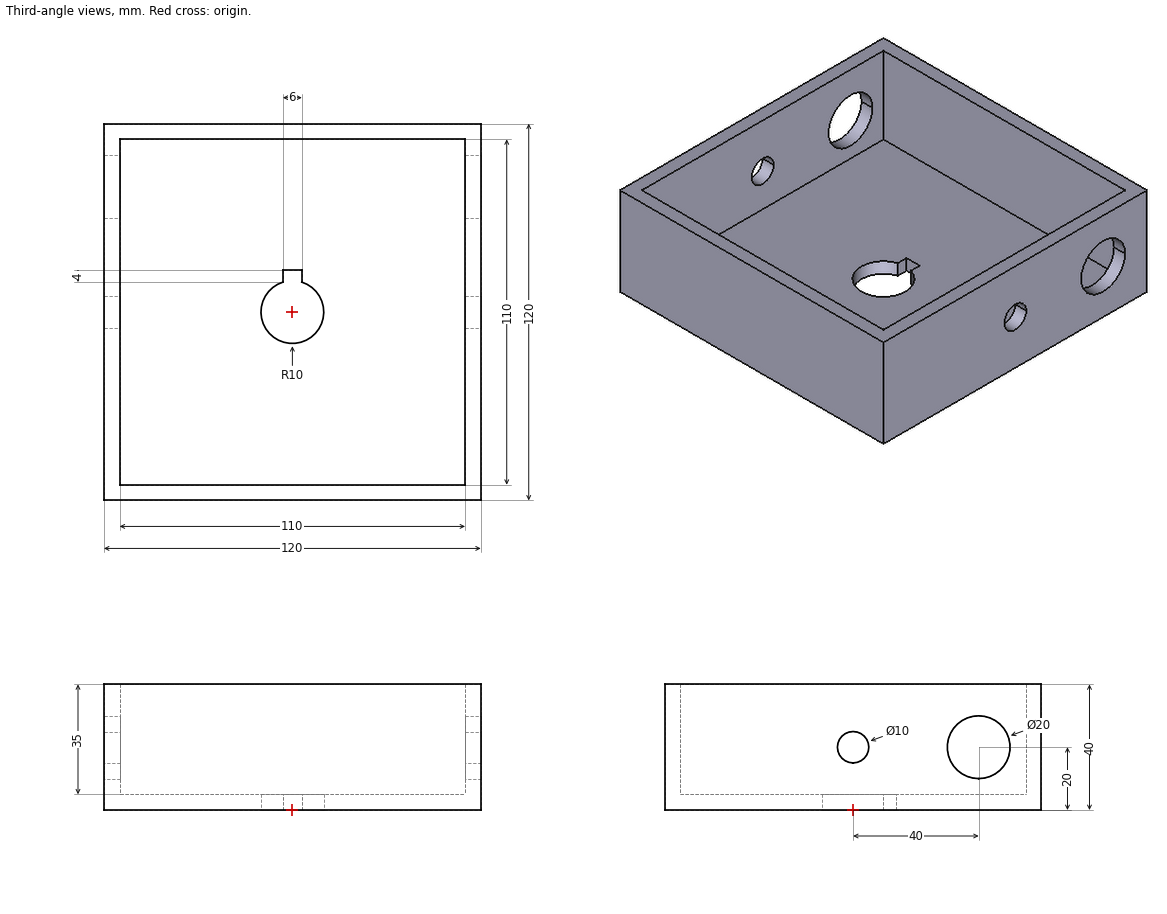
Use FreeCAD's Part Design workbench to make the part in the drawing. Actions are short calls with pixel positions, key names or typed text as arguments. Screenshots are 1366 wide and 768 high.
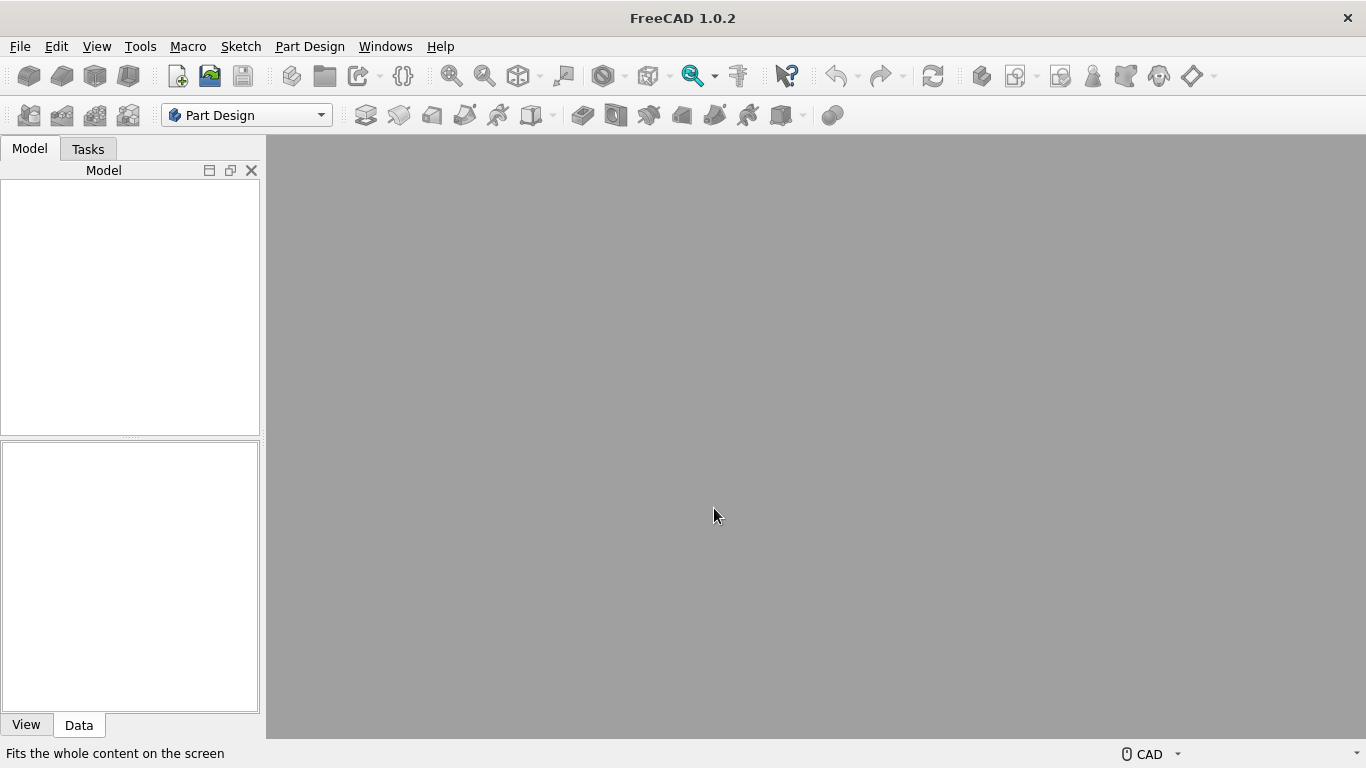
click(177, 76)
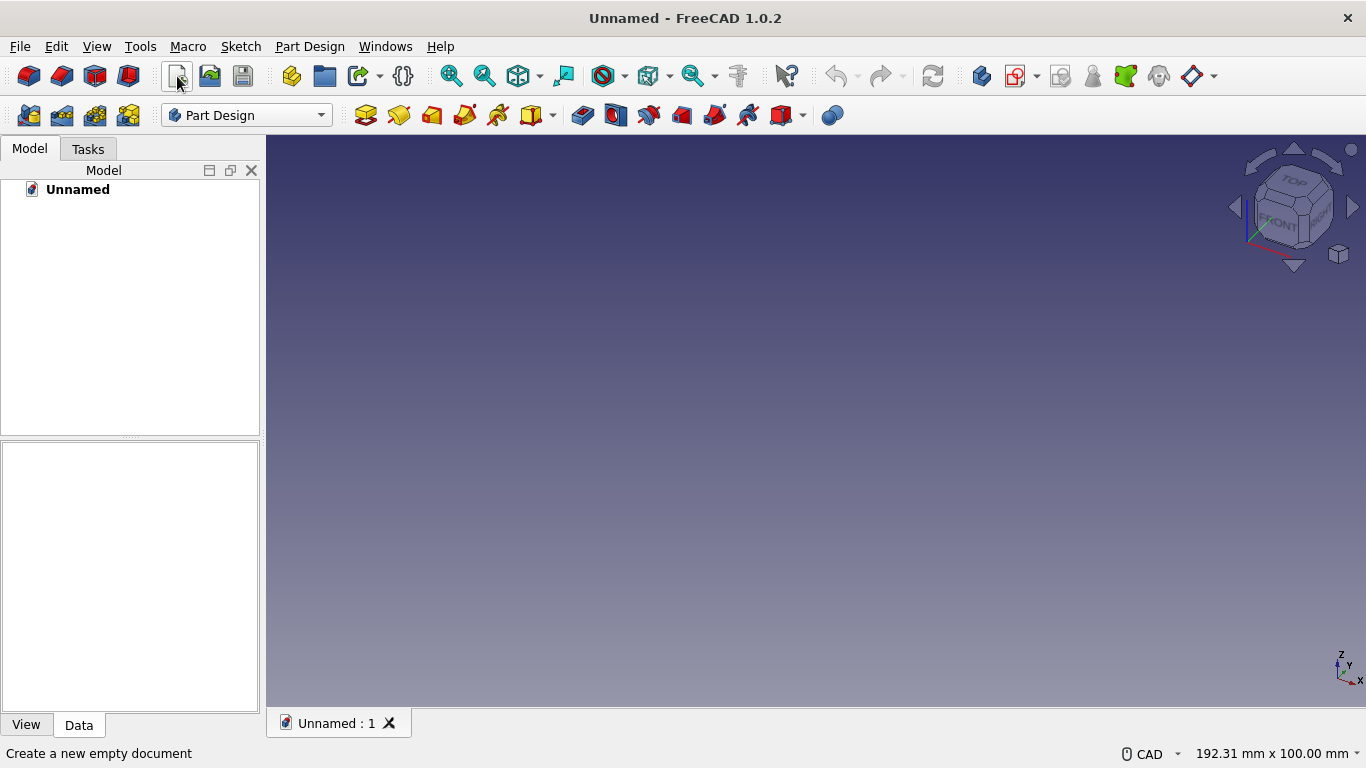
click(1014, 76)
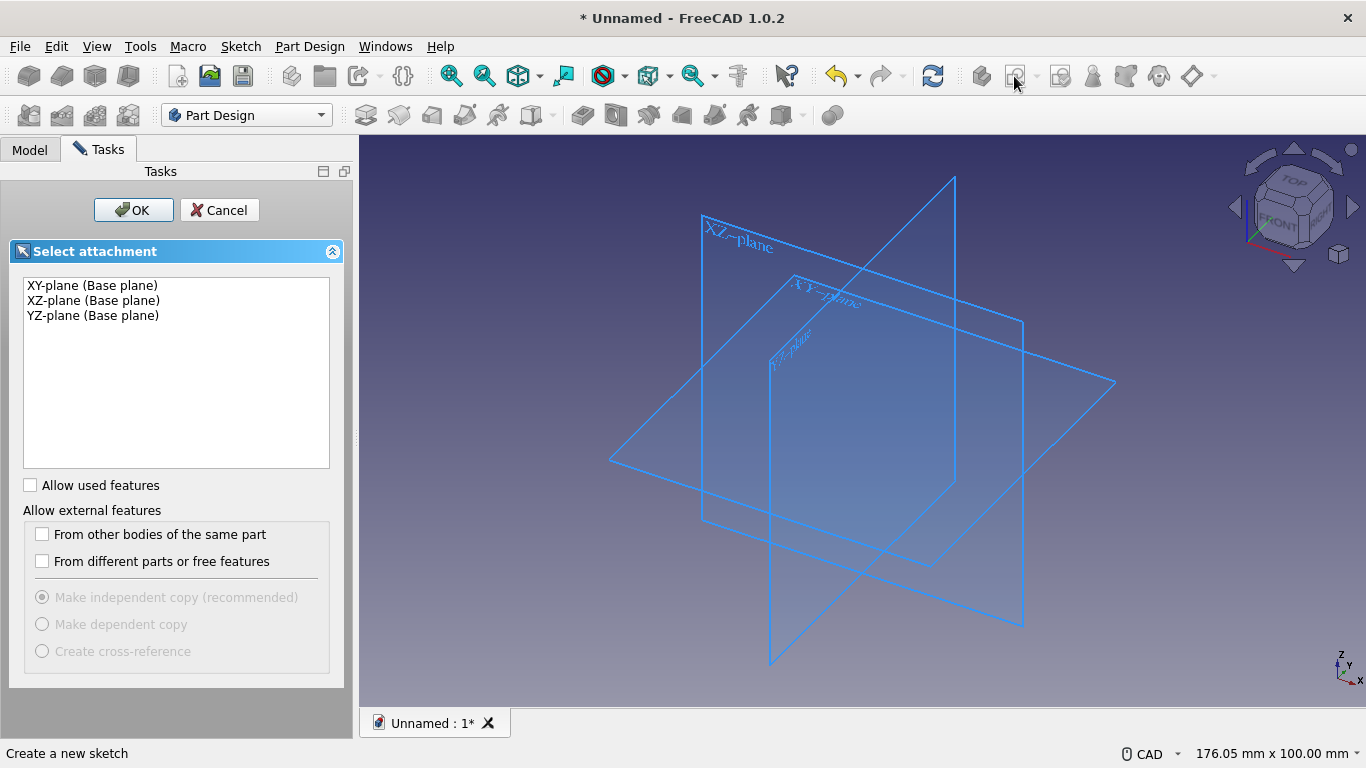
click(84, 286)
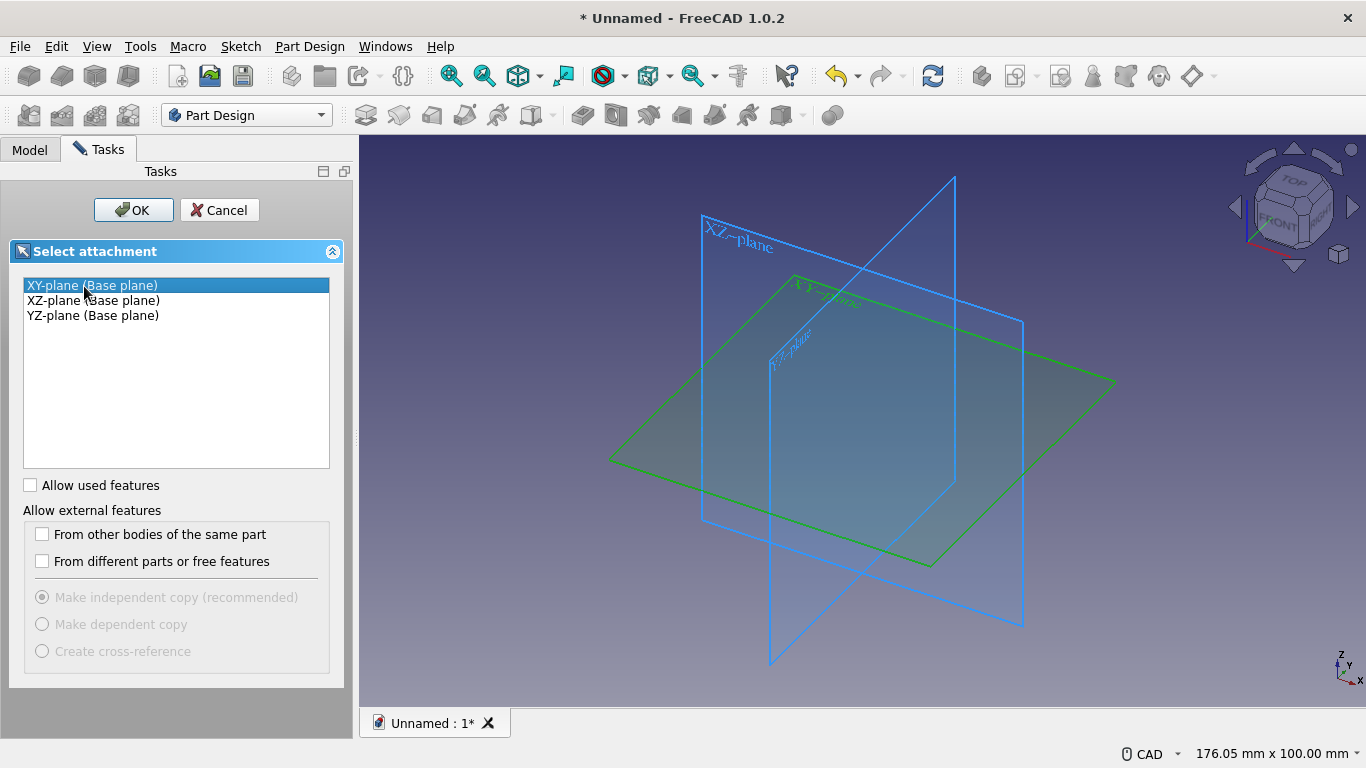
click(134, 210)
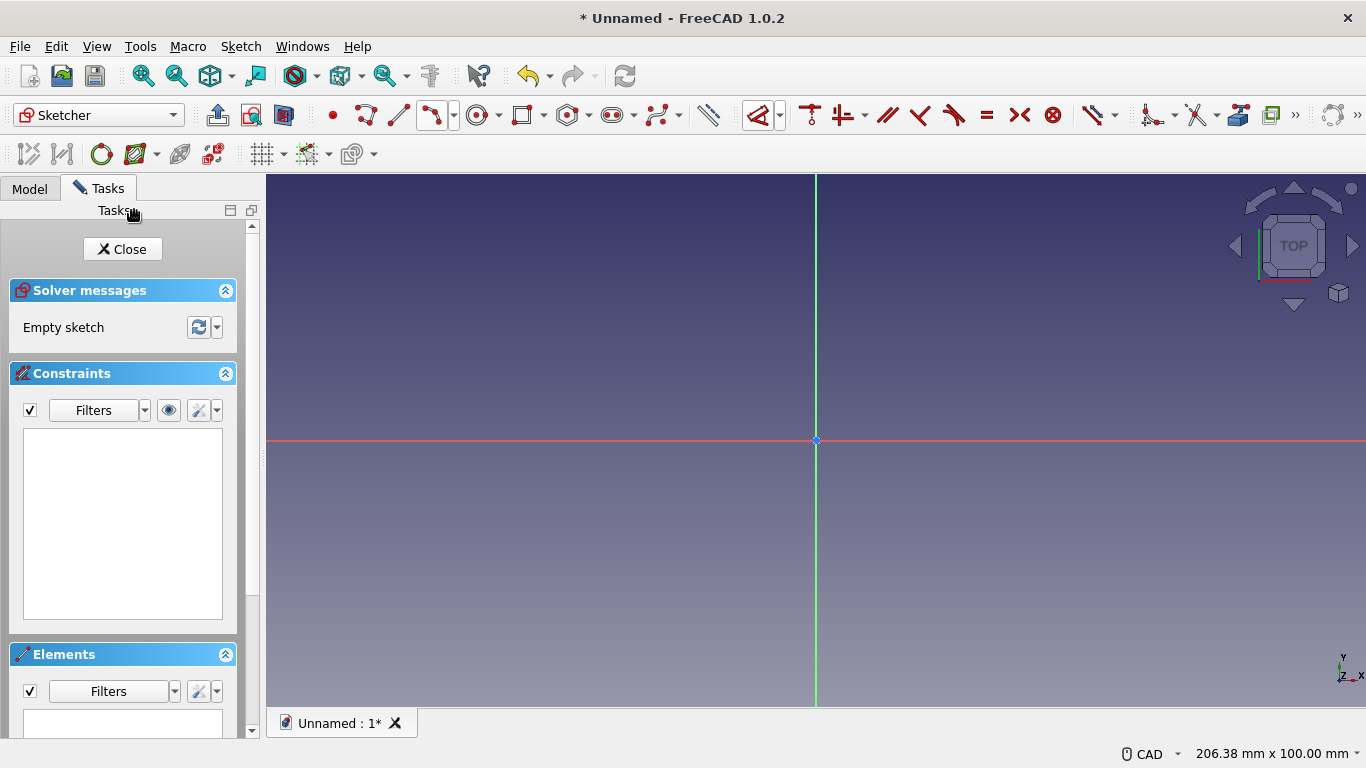
scroll(664, 440, down, 3)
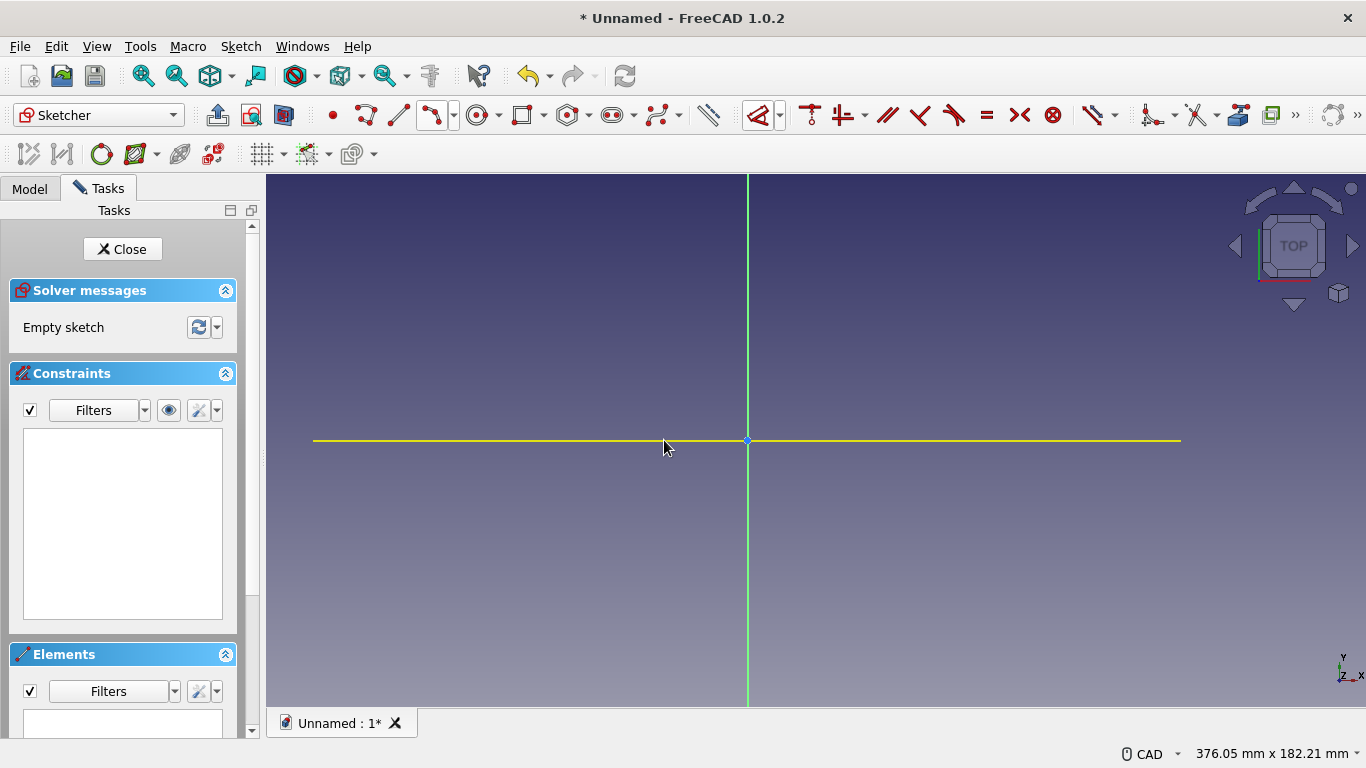
key(g)
key(v)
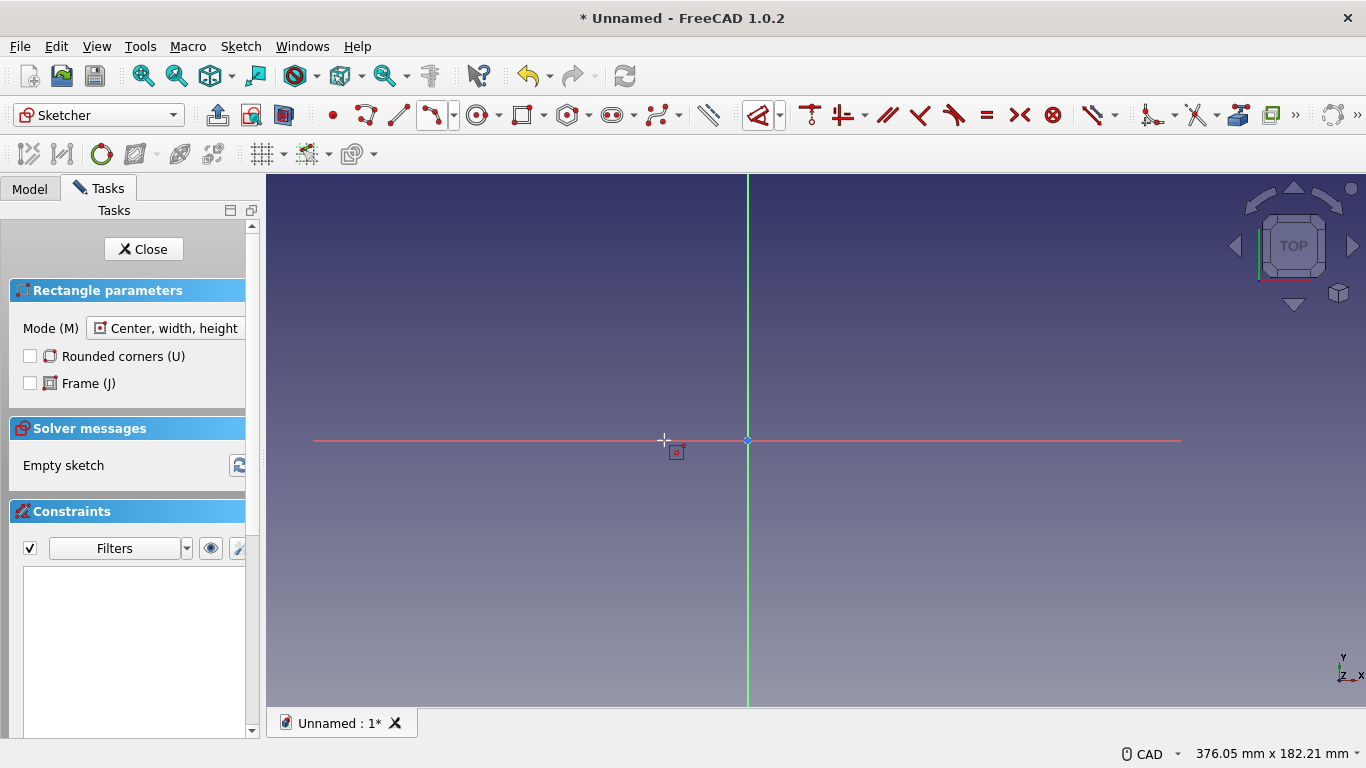
click(748, 440)
move(923, 265)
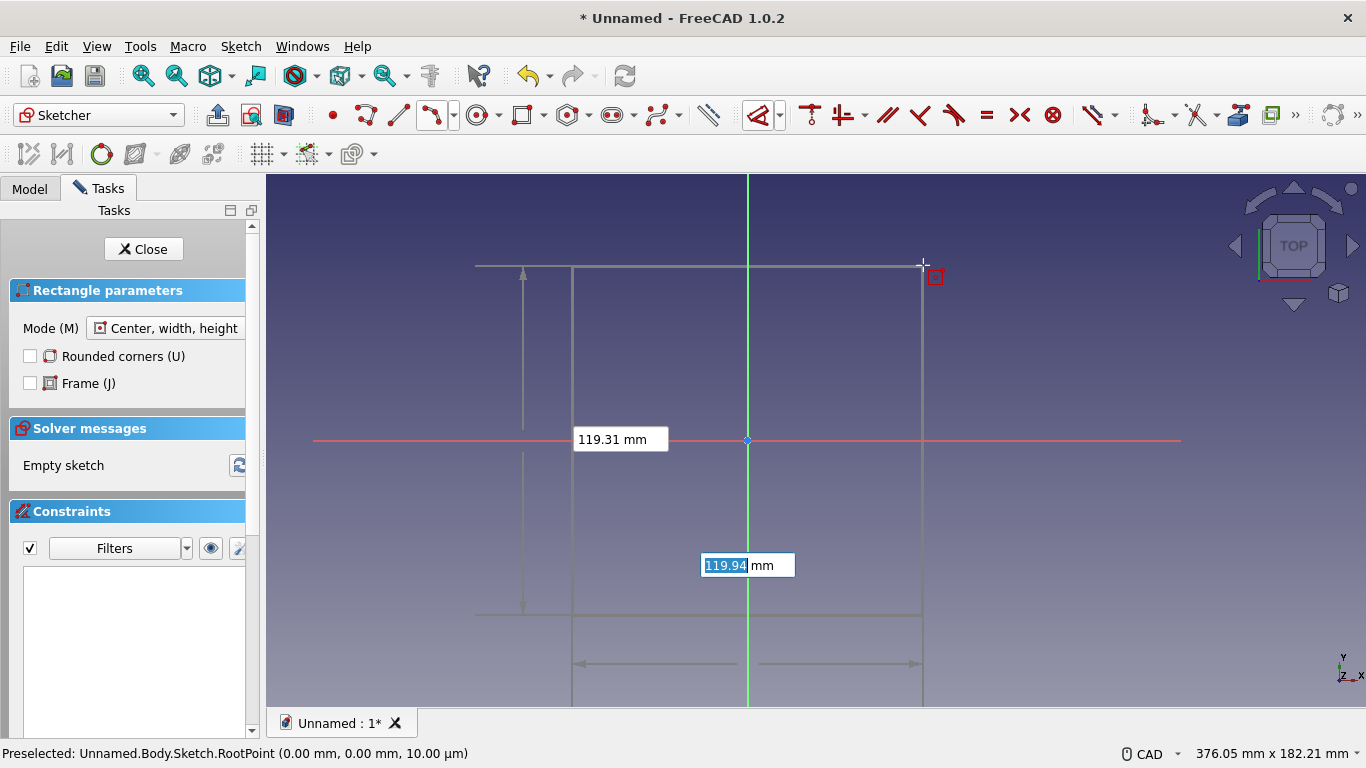
text(120)
key(Tab)
text(120)
key(Return)
key(Escape)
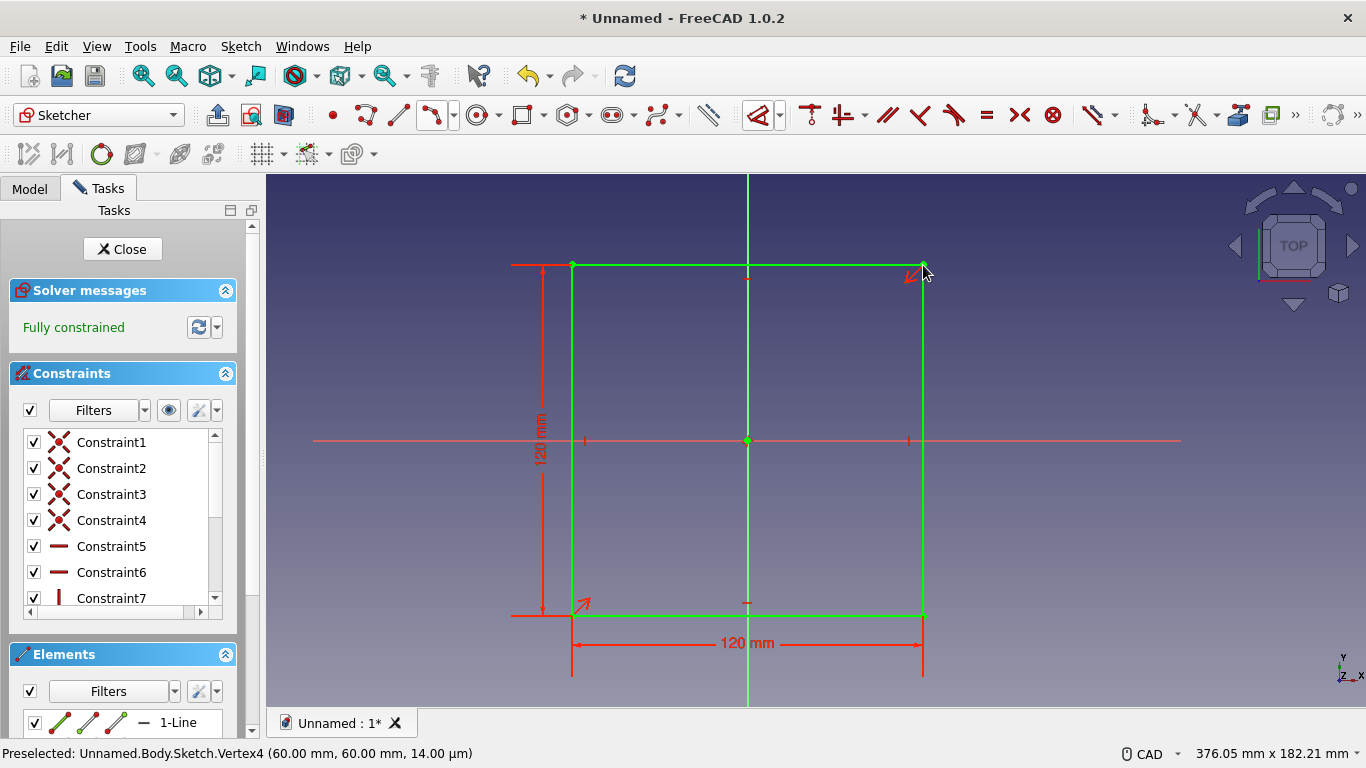
click(123, 249)